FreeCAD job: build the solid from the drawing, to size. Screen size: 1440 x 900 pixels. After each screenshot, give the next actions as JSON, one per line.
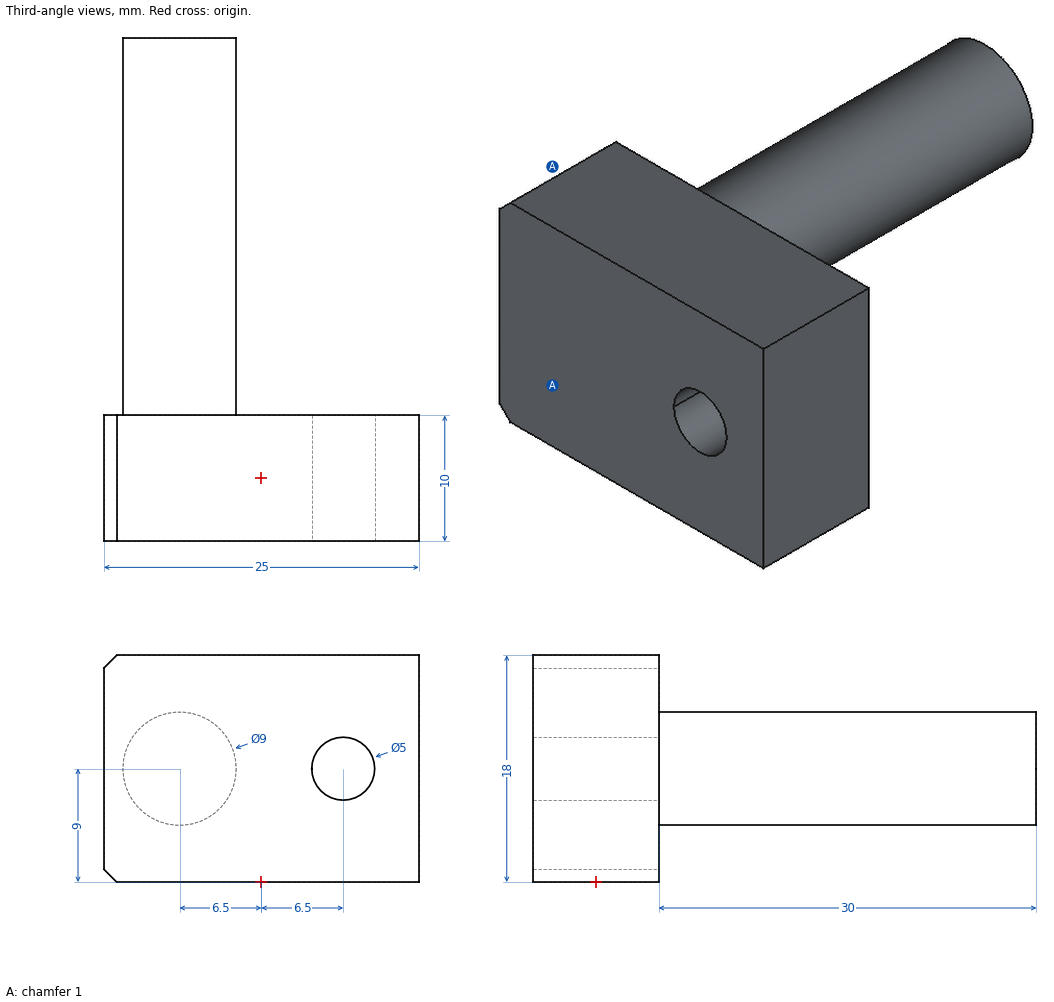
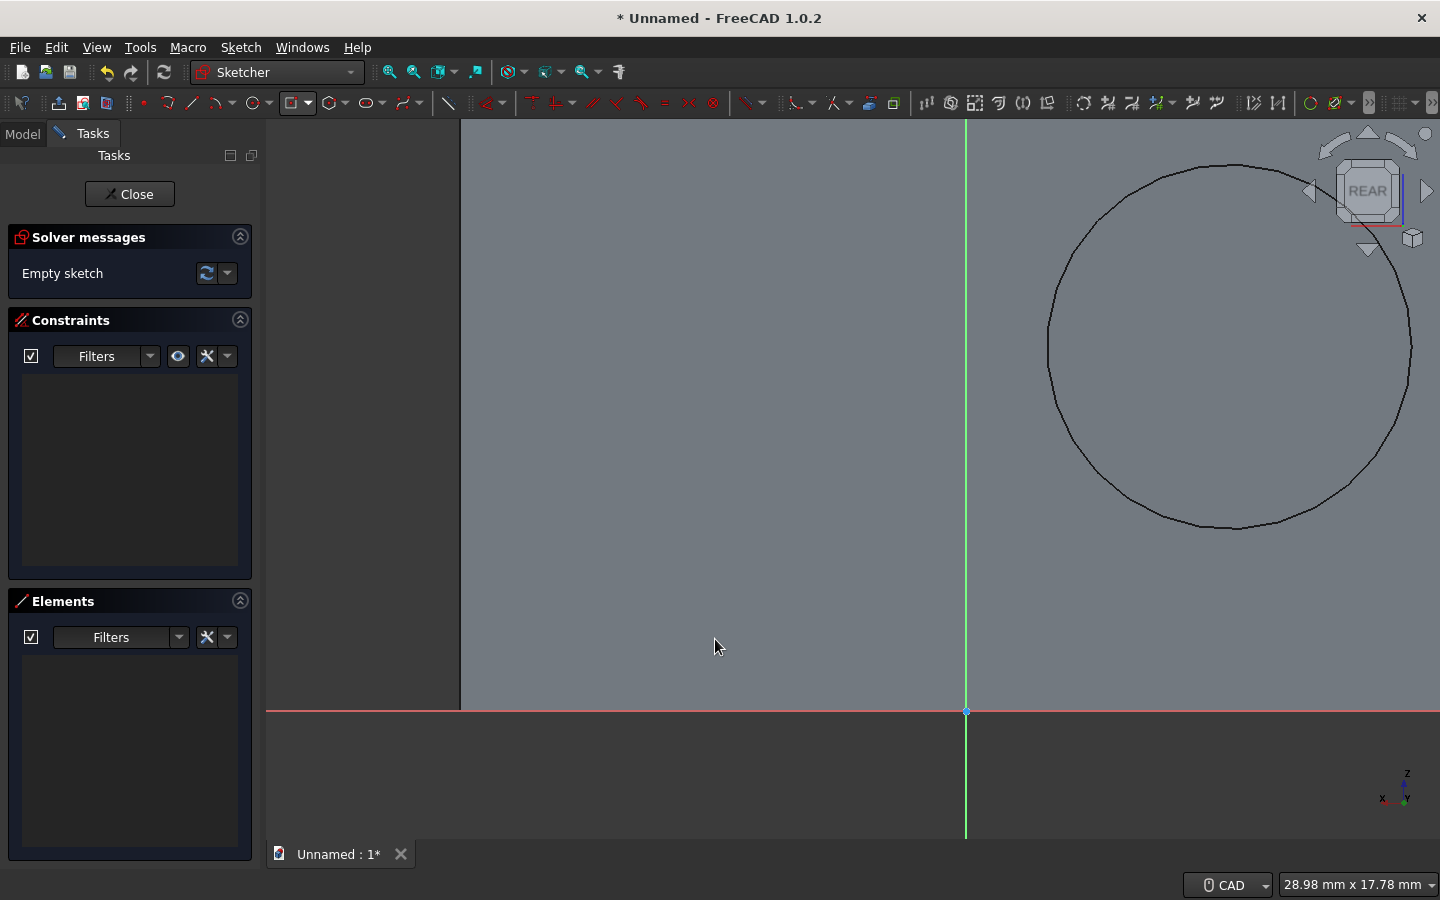
{"action": "key", "text": "g c"}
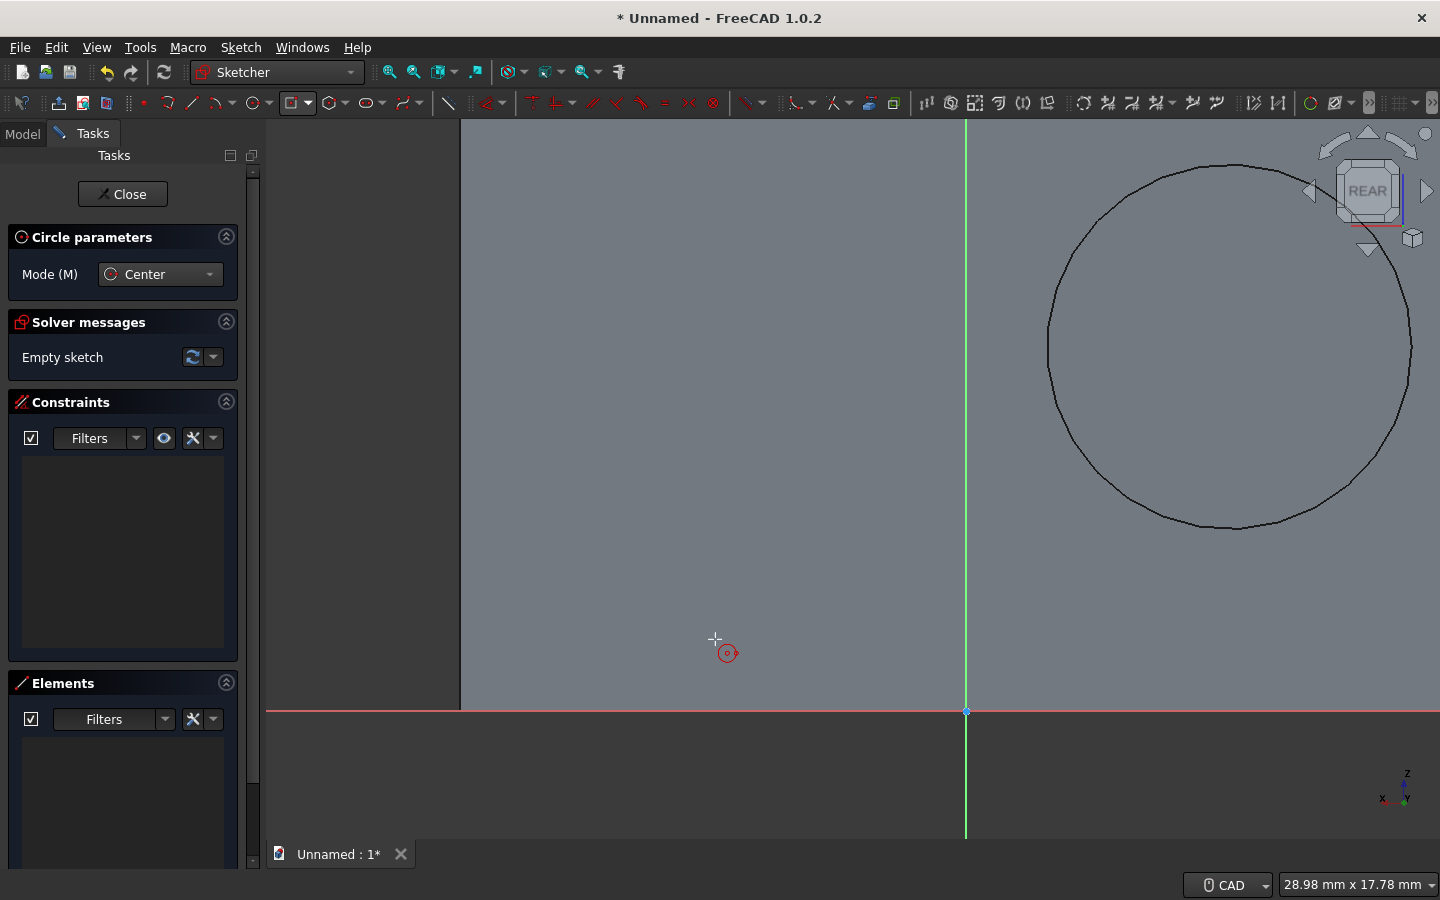
{"action": "left_click", "coordinate": [703, 347]}
{"action": "mouse_move", "coordinate": [774, 275]}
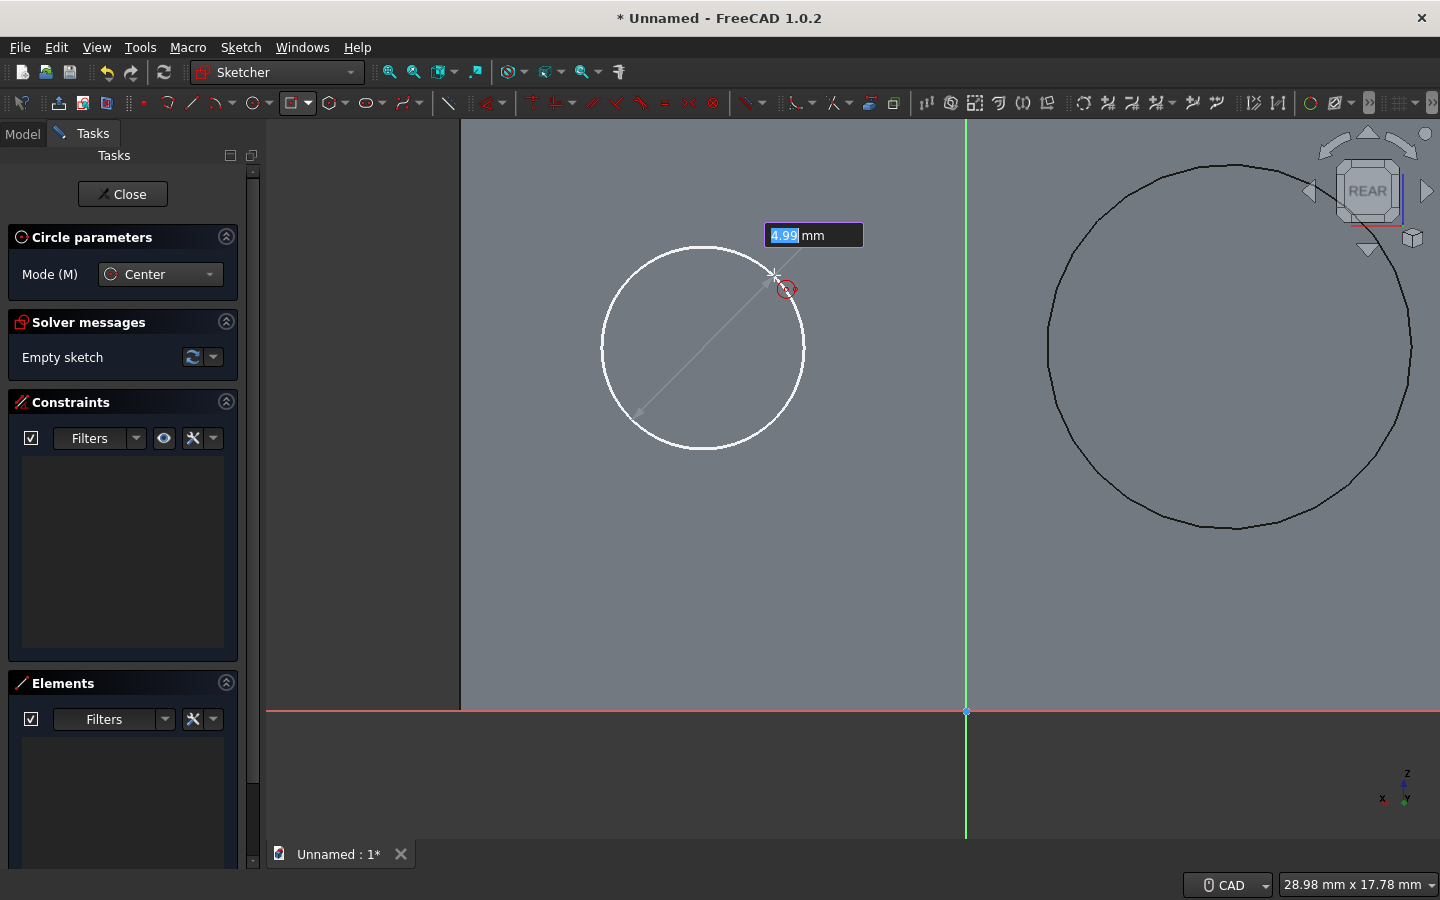
{"action": "type", "text": "5"}
{"action": "key", "text": "Return"}
{"action": "key", "text": "Escape"}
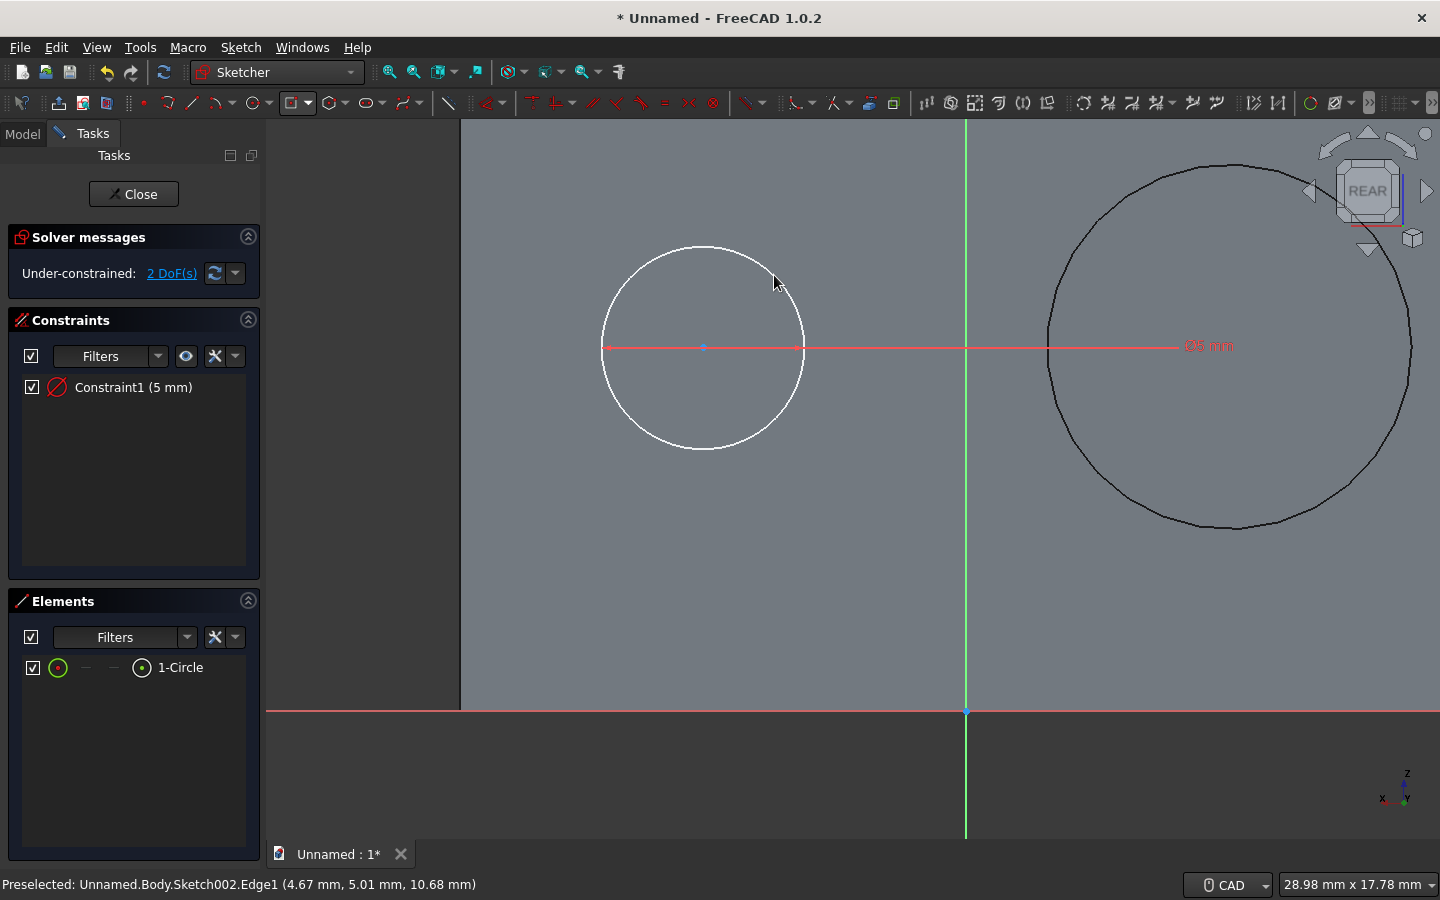
{"action": "left_click", "coordinate": [703, 348]}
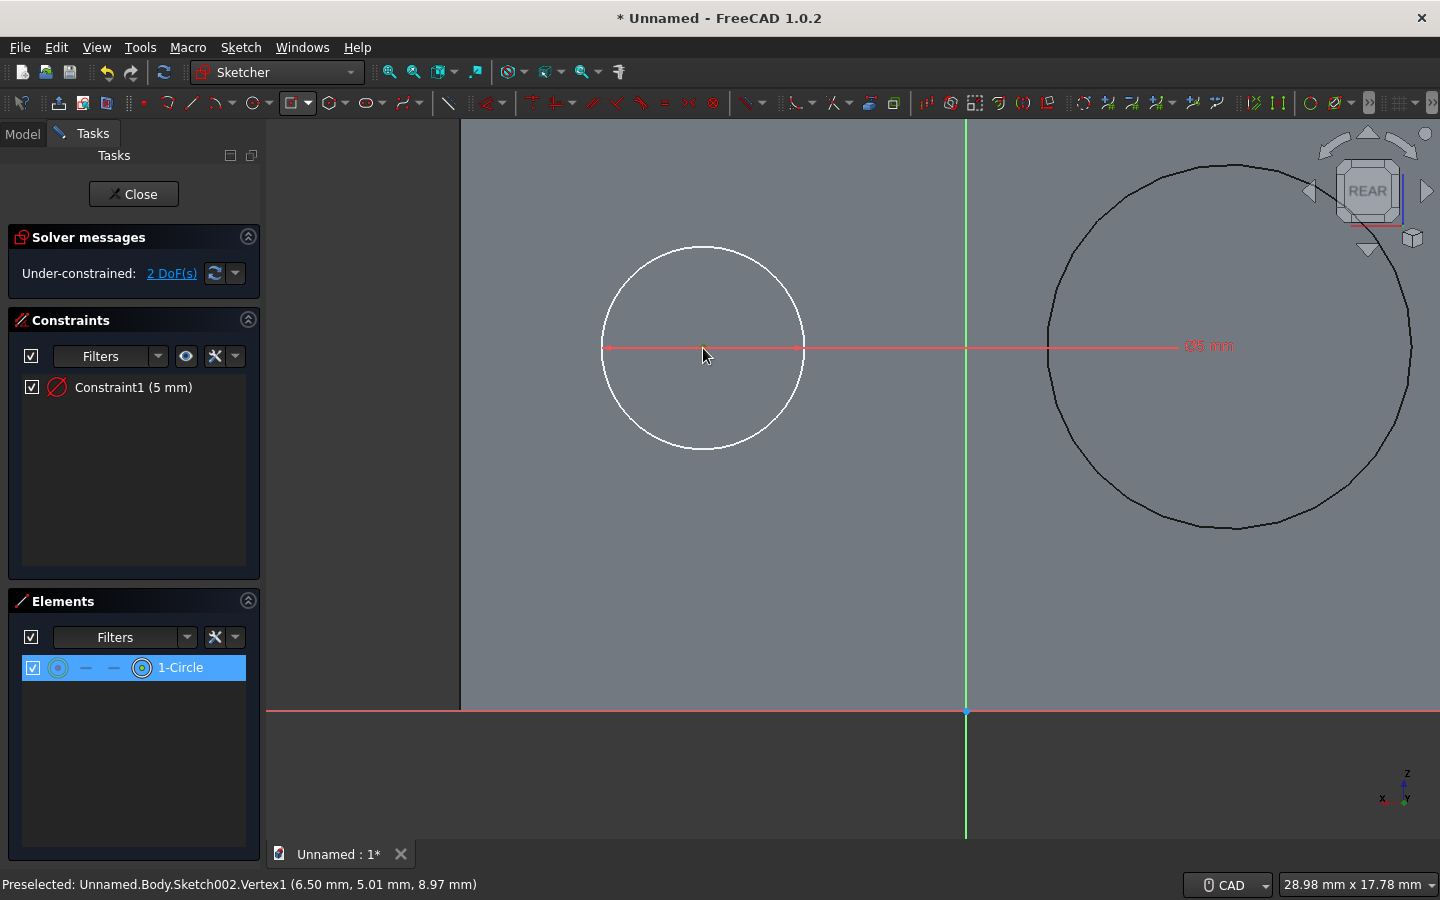
{"action": "left_click", "coordinate": [504, 104]}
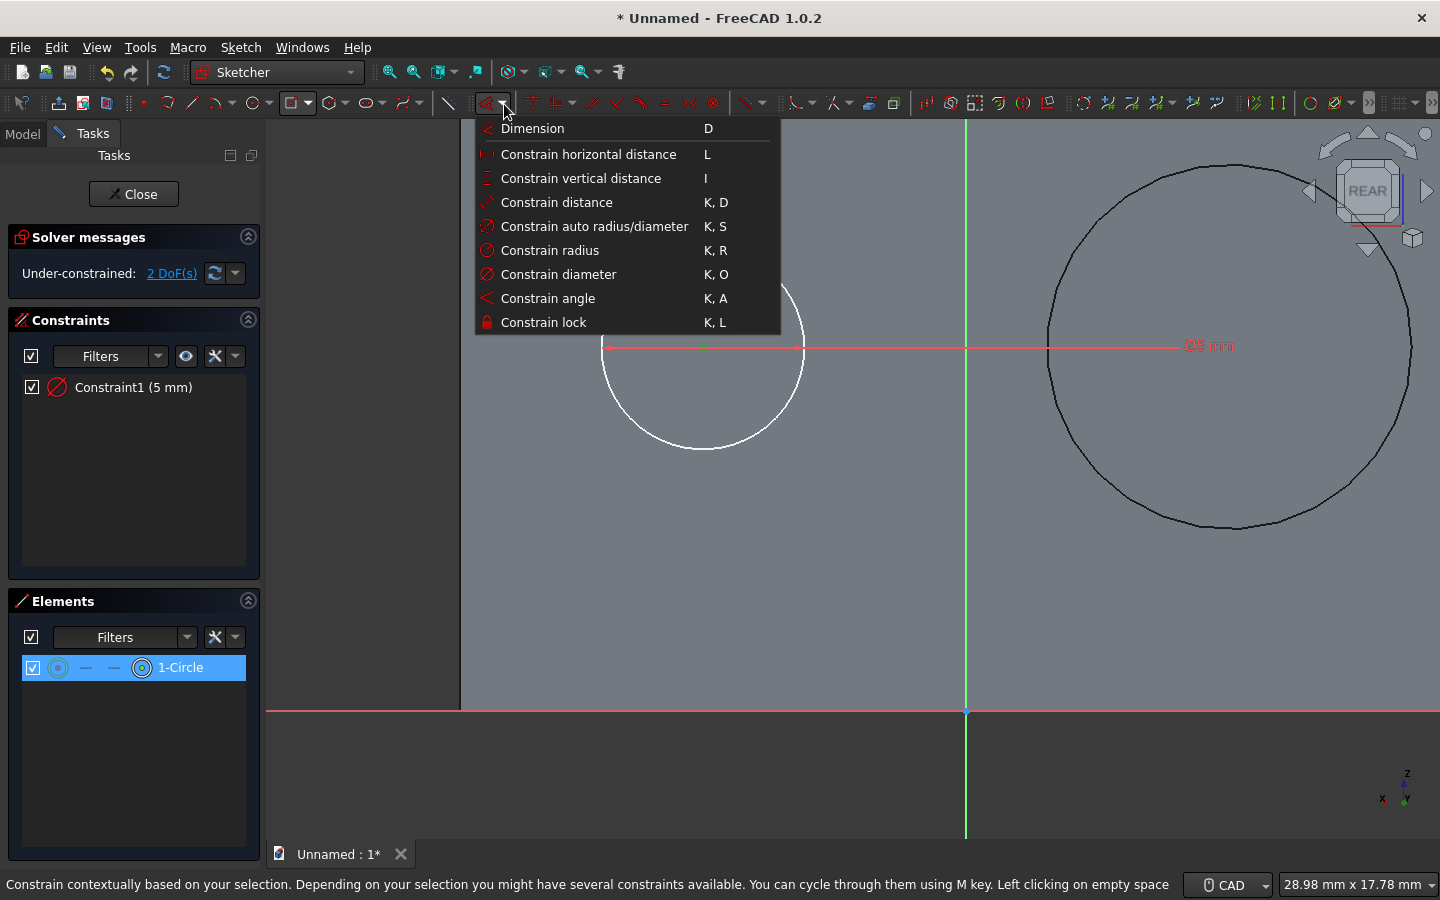
{"action": "left_click", "coordinate": [628, 178]}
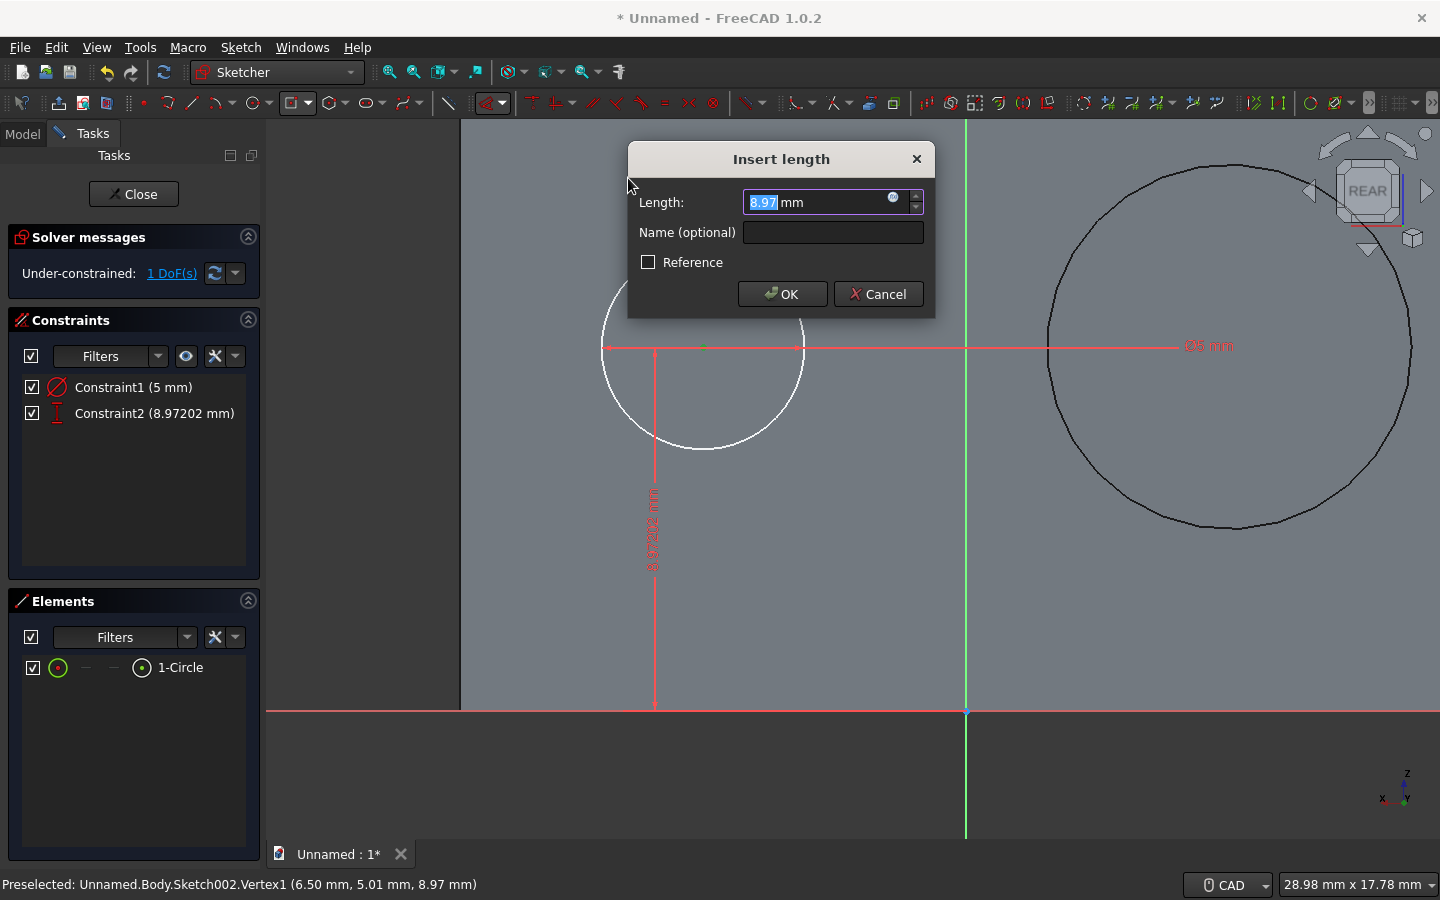
{"action": "type", "text": "9"}
{"action": "key", "text": "Return"}